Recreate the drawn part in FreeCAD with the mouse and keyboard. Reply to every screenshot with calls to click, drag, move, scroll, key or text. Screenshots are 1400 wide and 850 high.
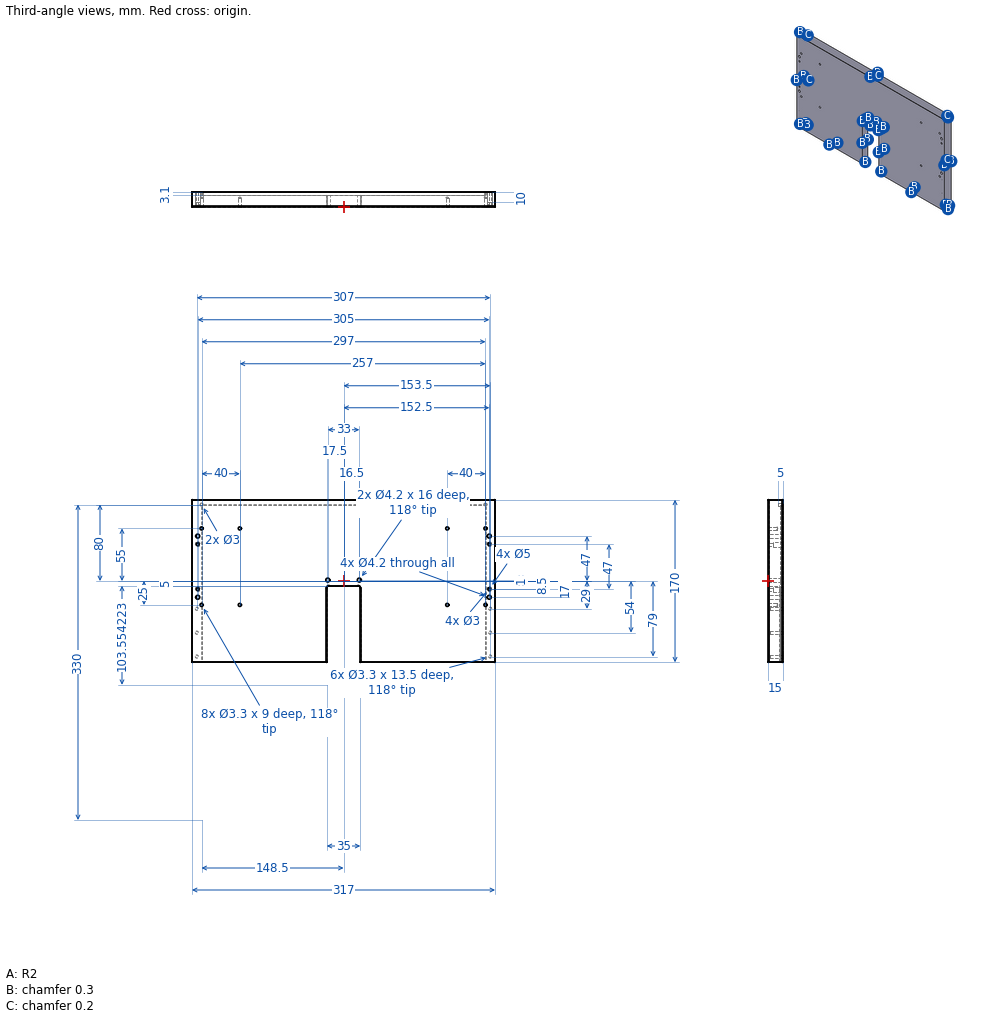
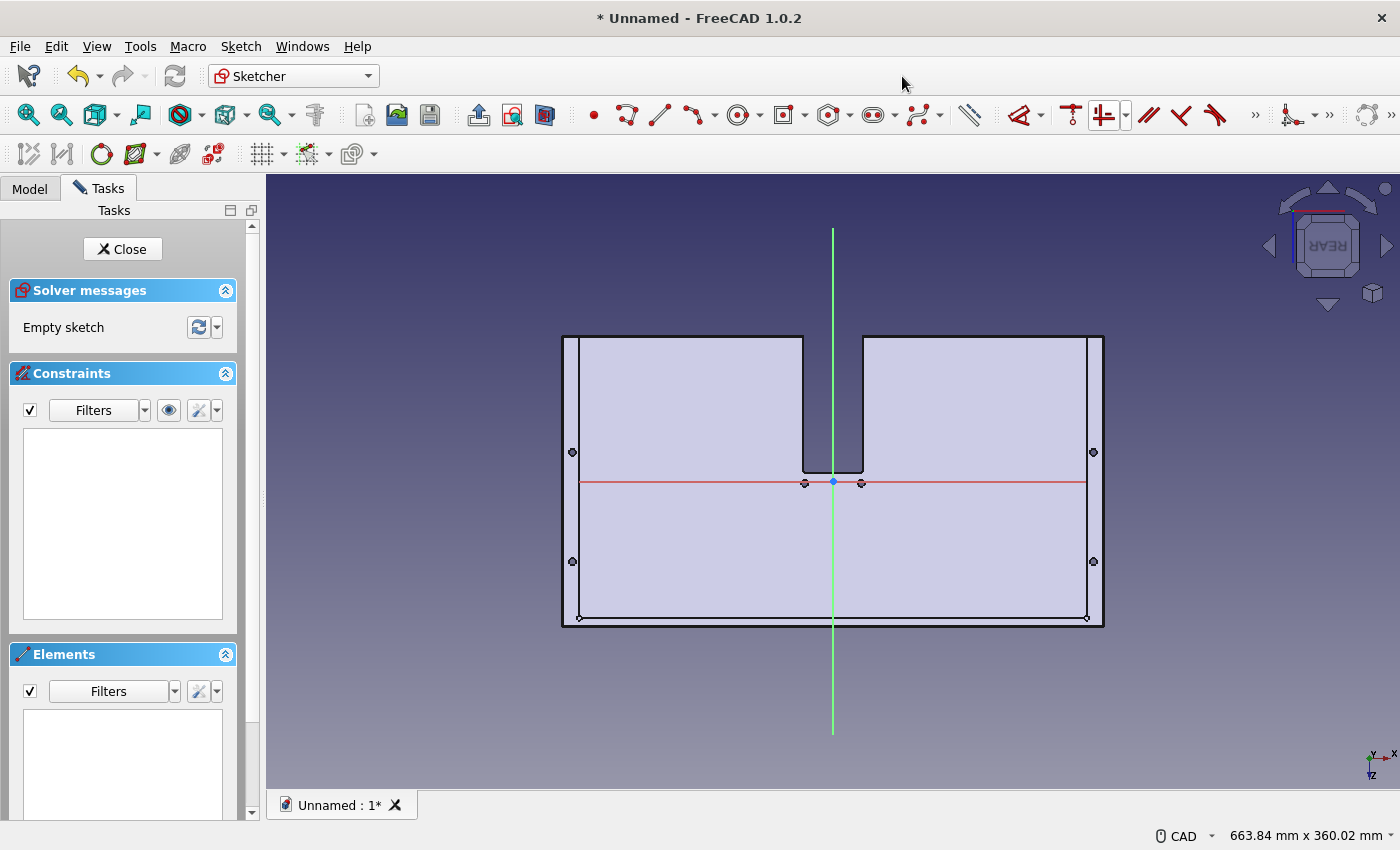
click(738, 116)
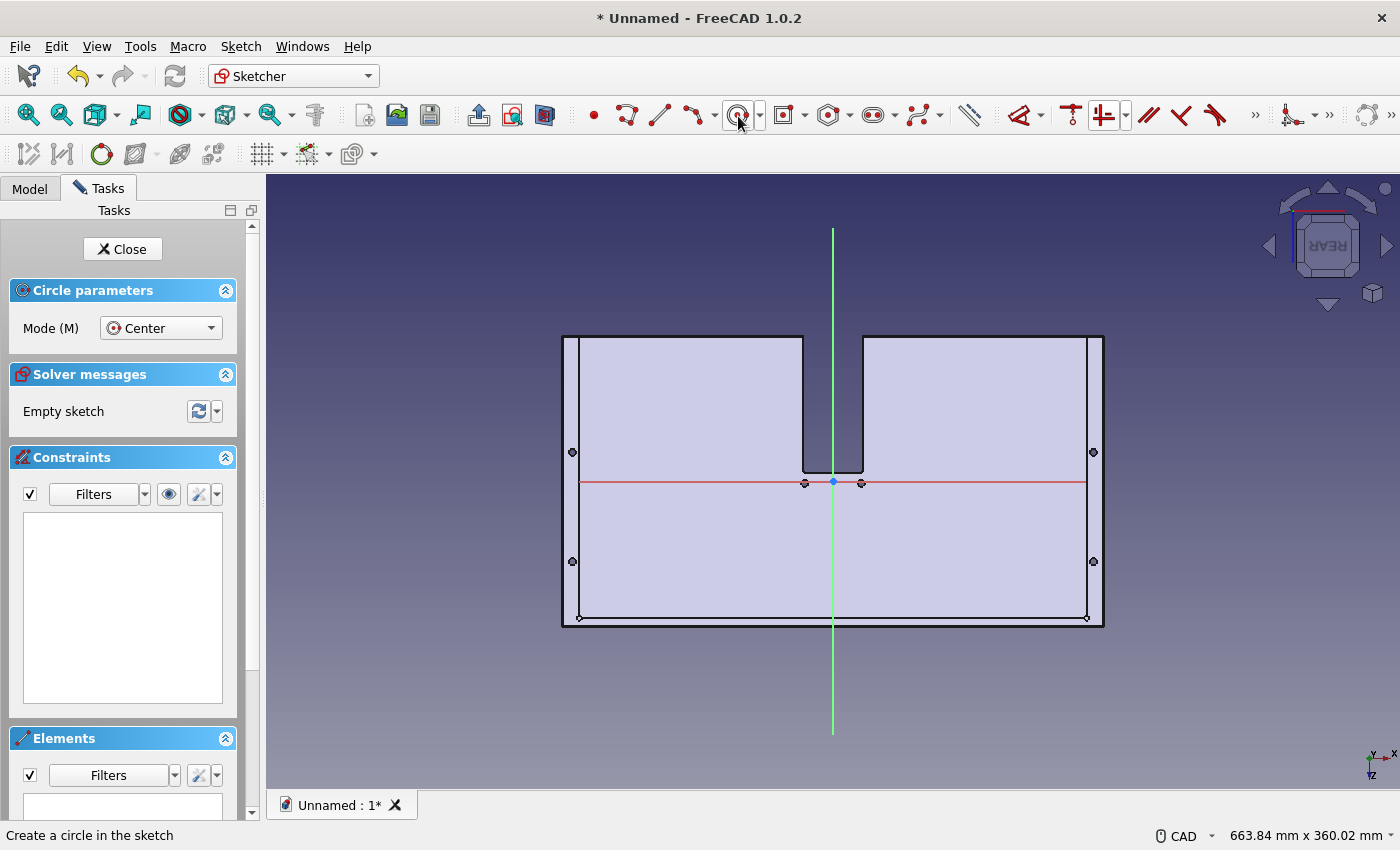
scroll(1095, 347, up, 11)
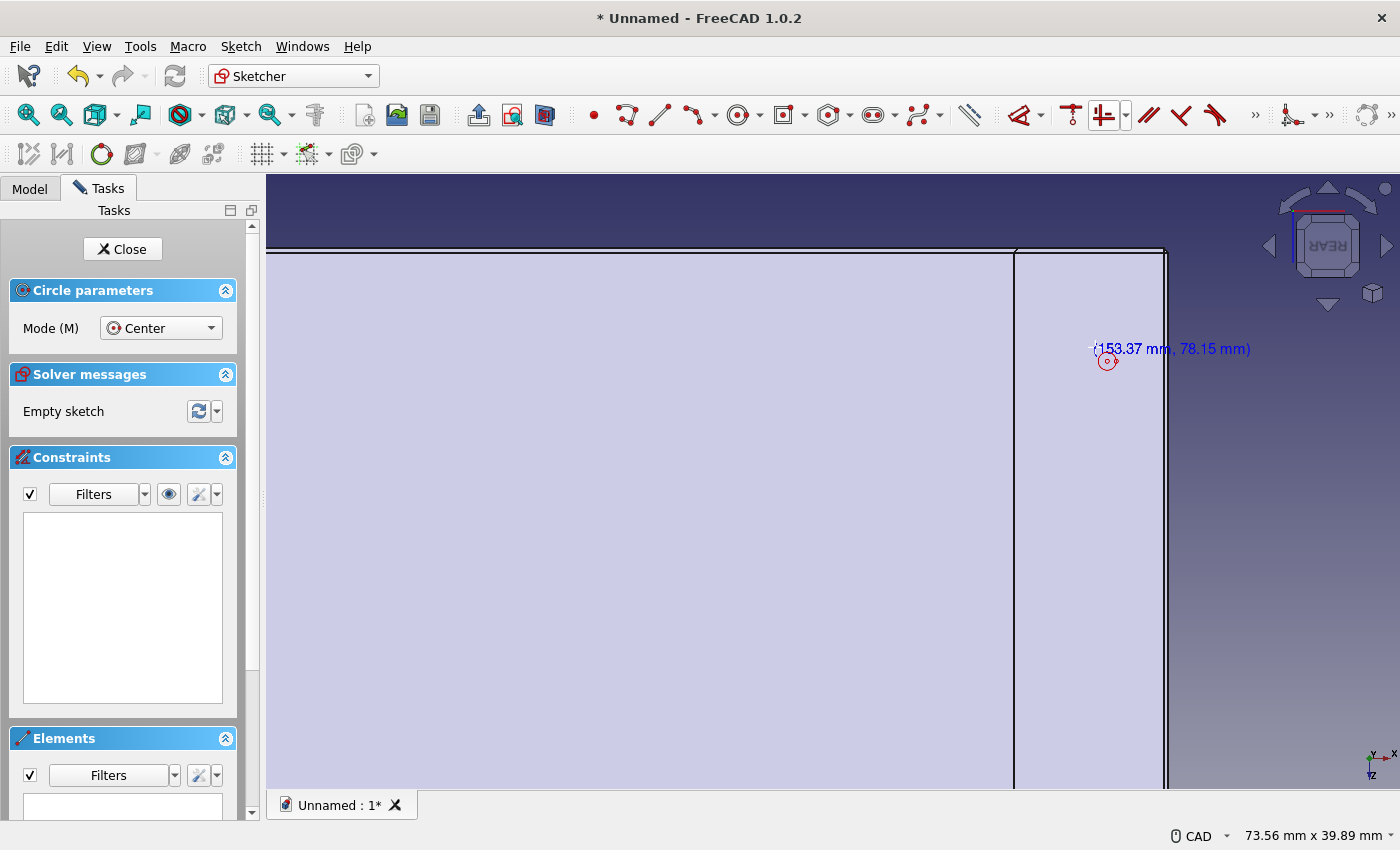
scroll(1084, 410, down, 10)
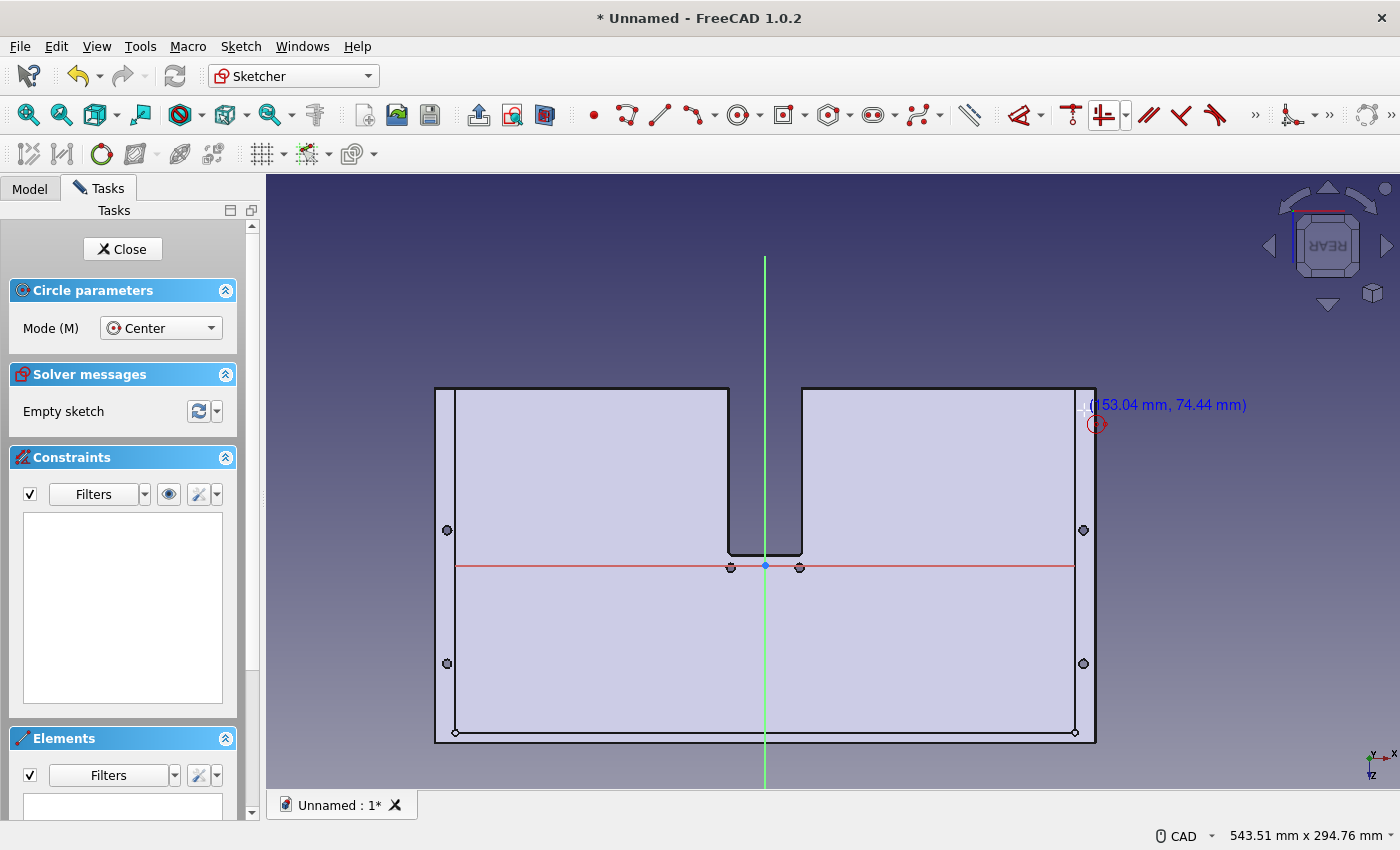
click(1086, 401)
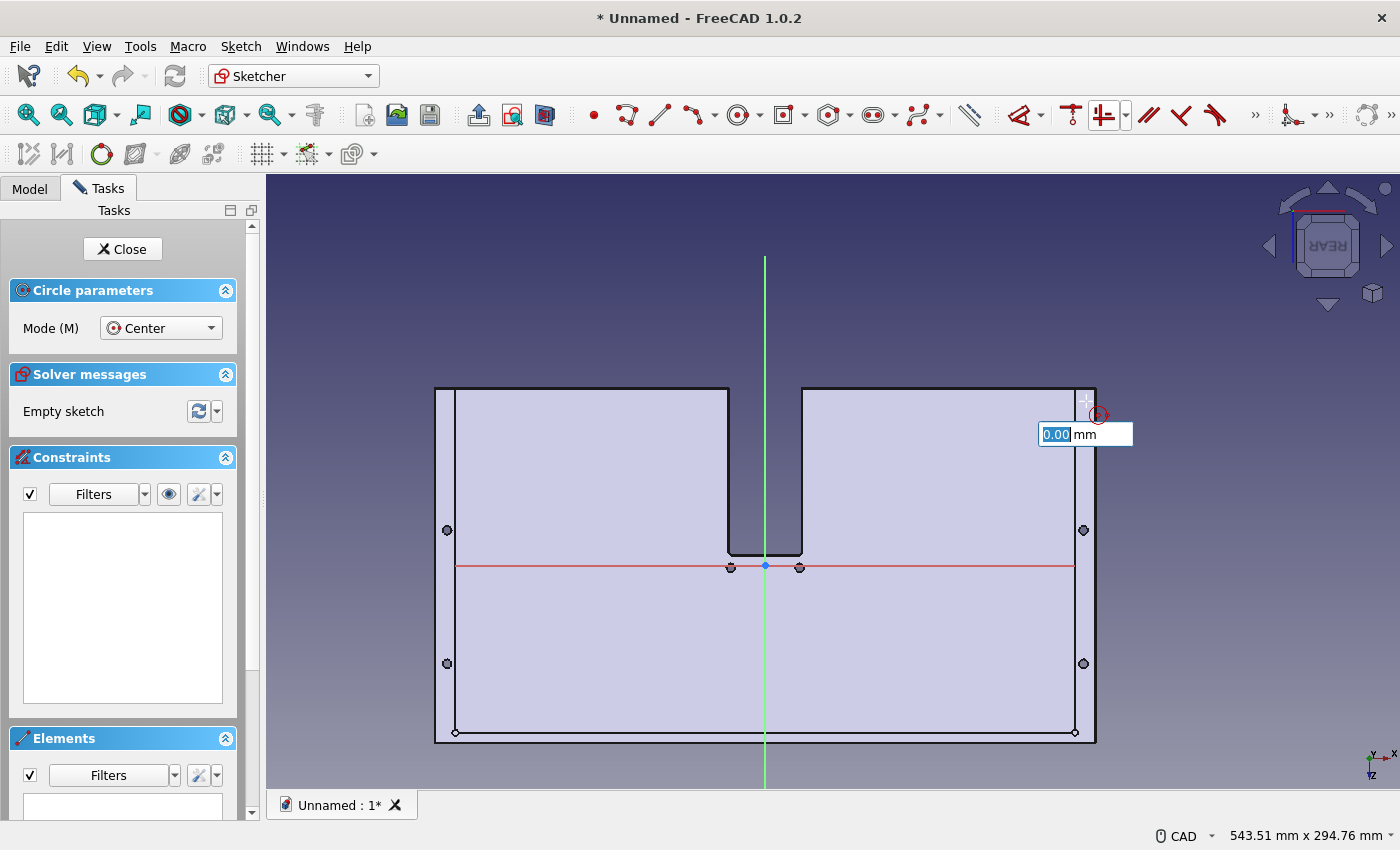
scroll(1088, 399, up, 8)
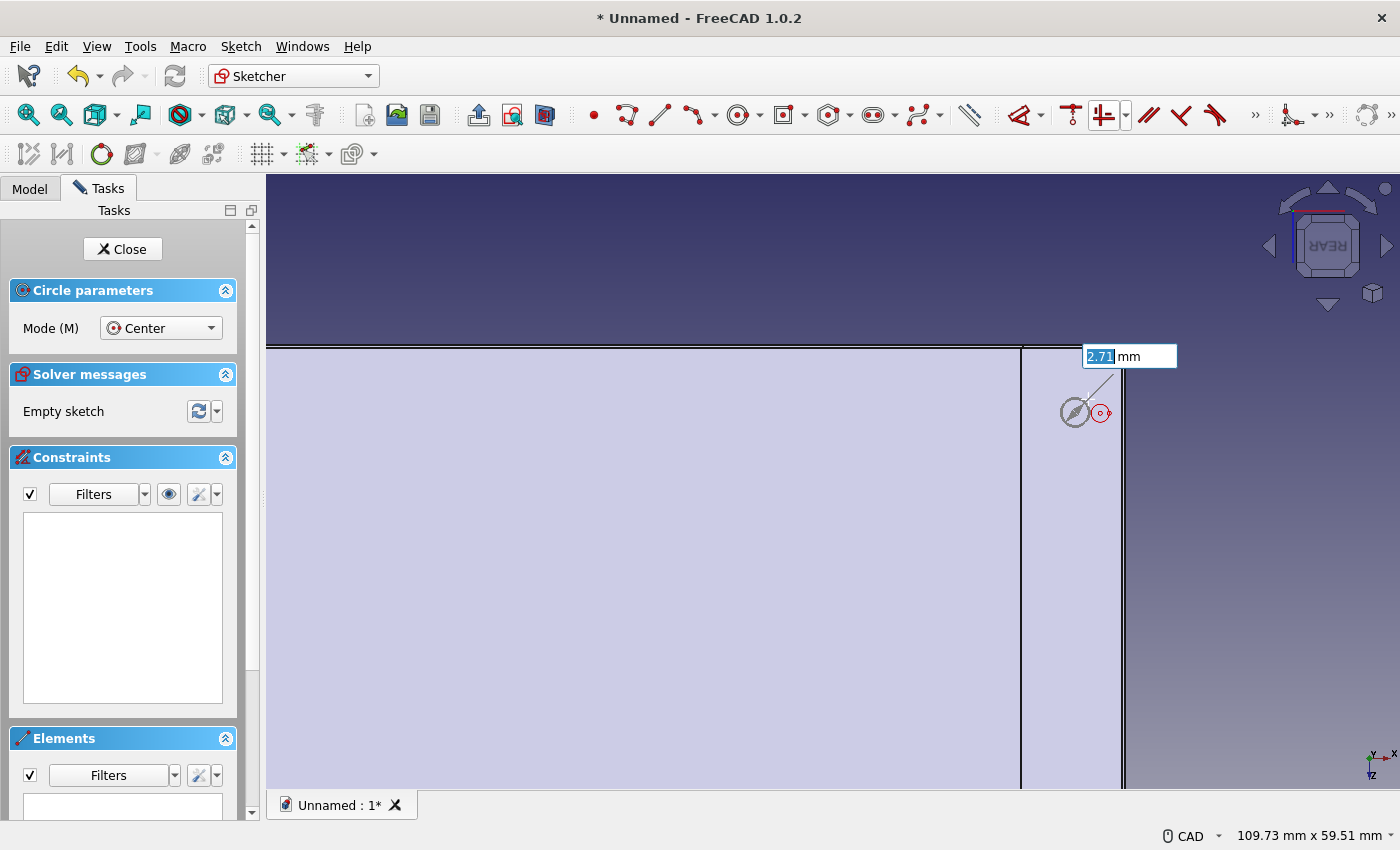
click(1085, 395)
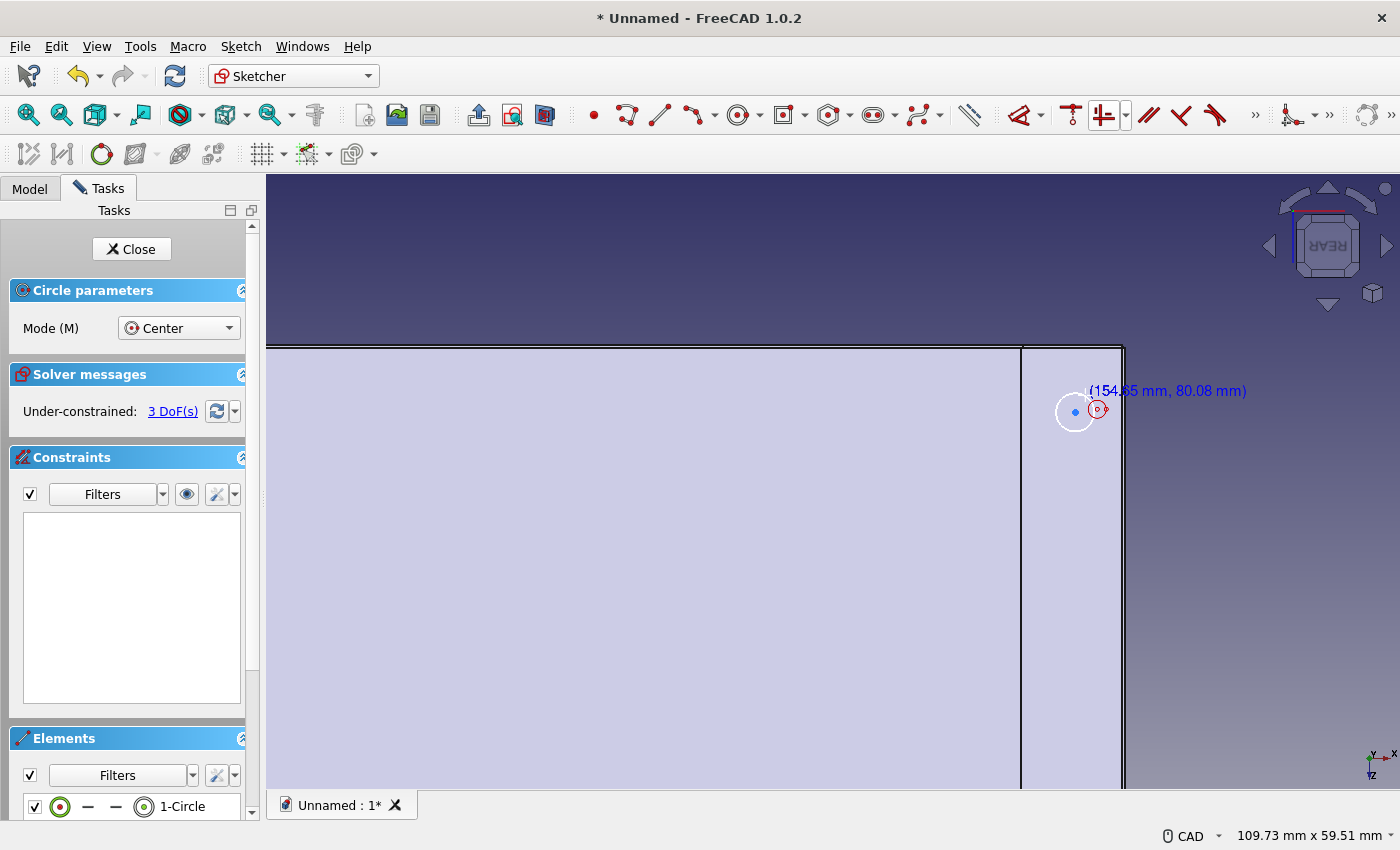
scroll(1073, 666, up, 2)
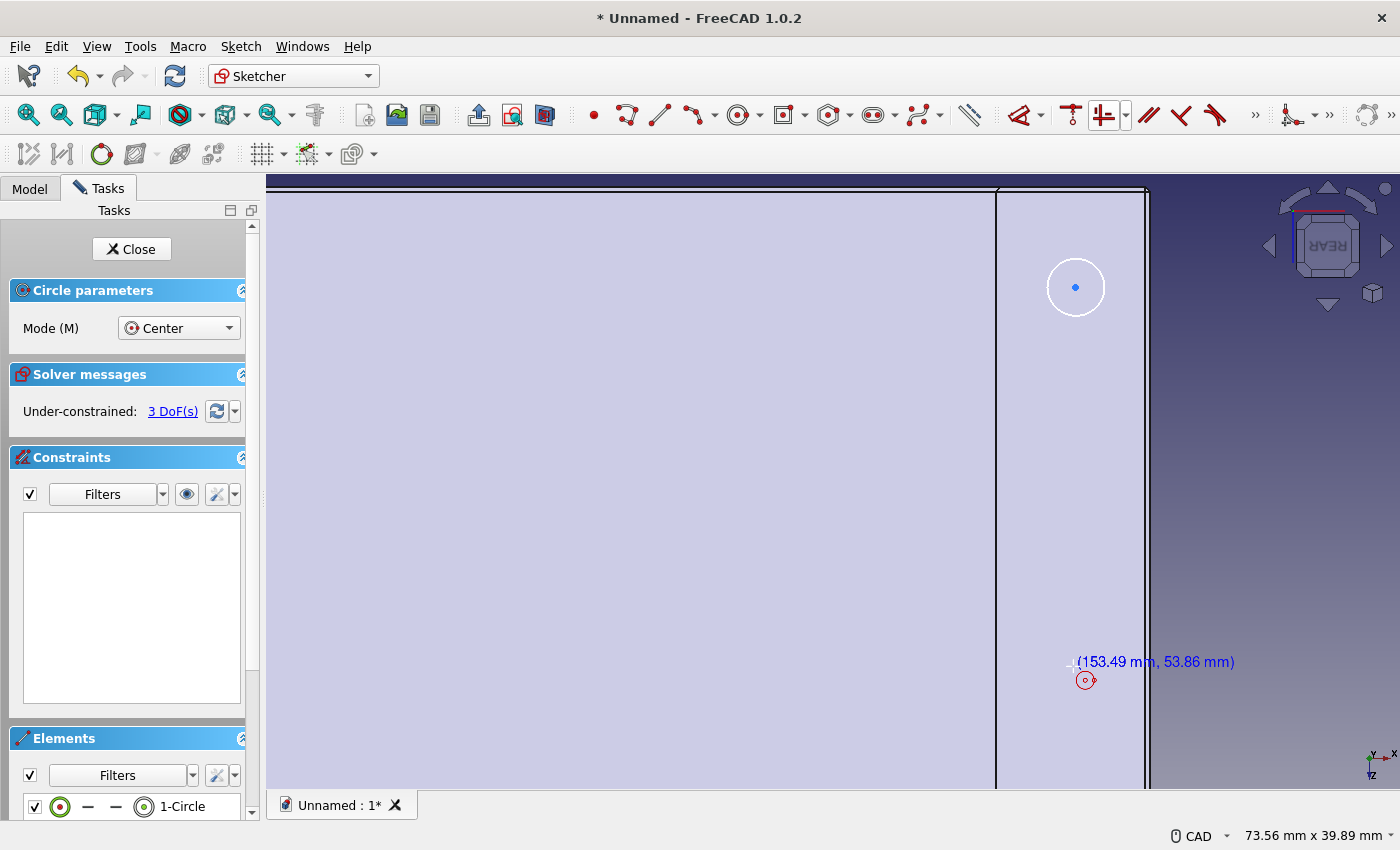
scroll(1087, 420, down, 10)